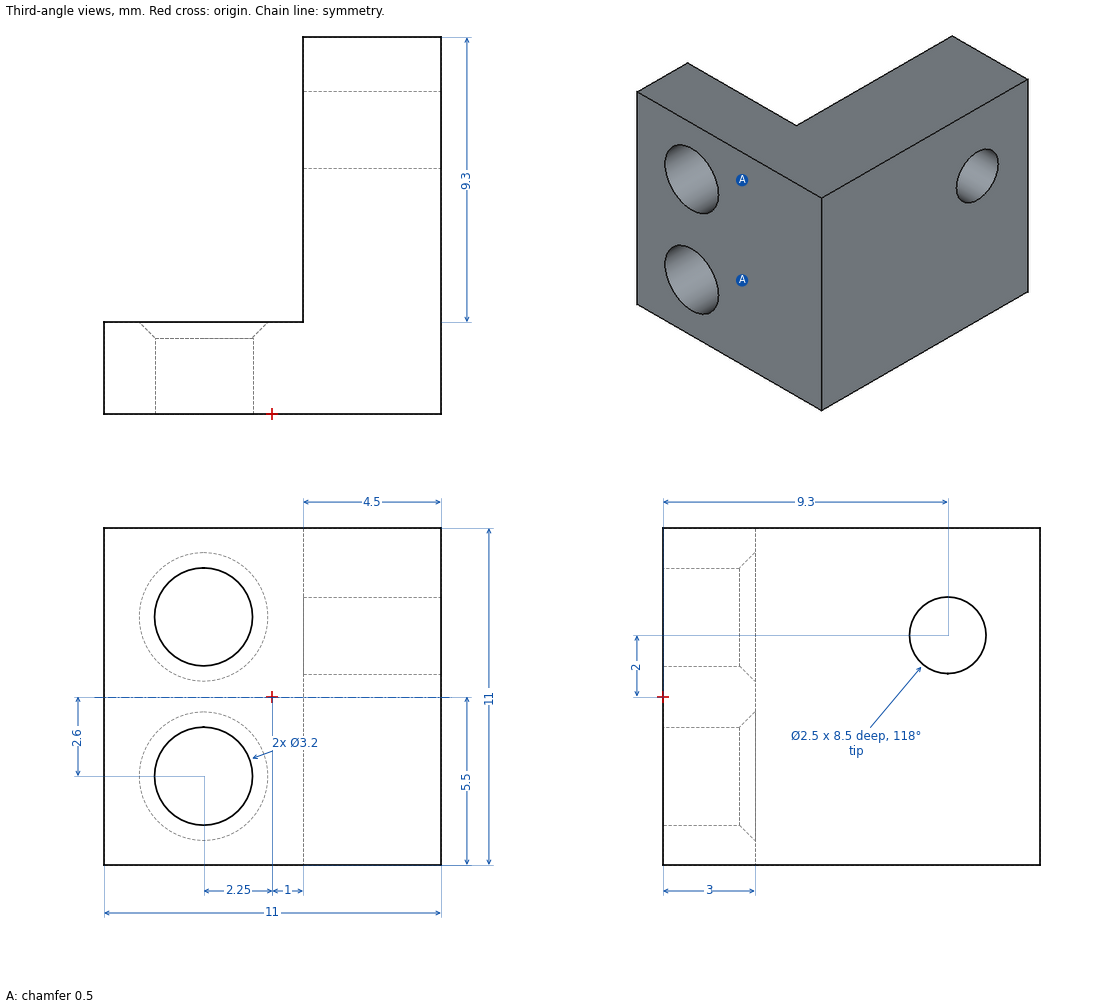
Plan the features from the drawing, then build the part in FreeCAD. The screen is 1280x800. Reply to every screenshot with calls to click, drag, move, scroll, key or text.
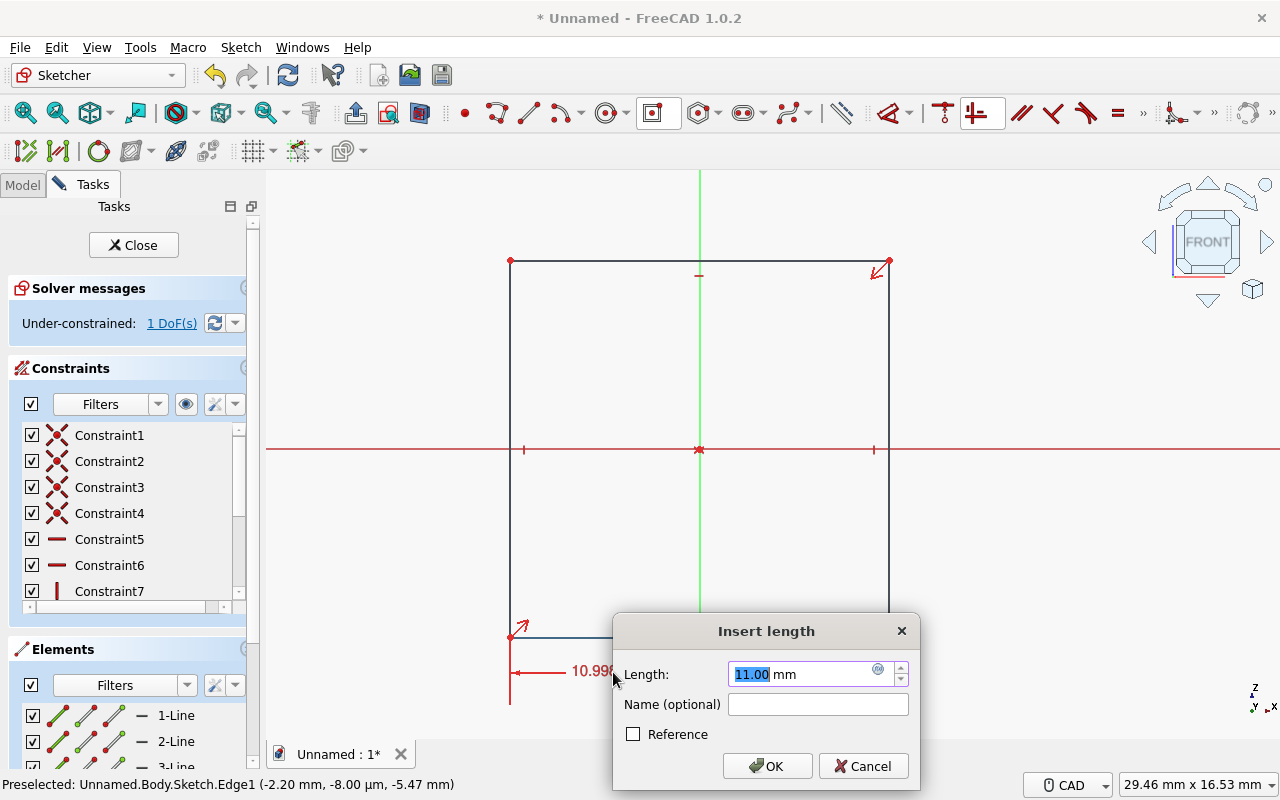
text(11)
key(Return)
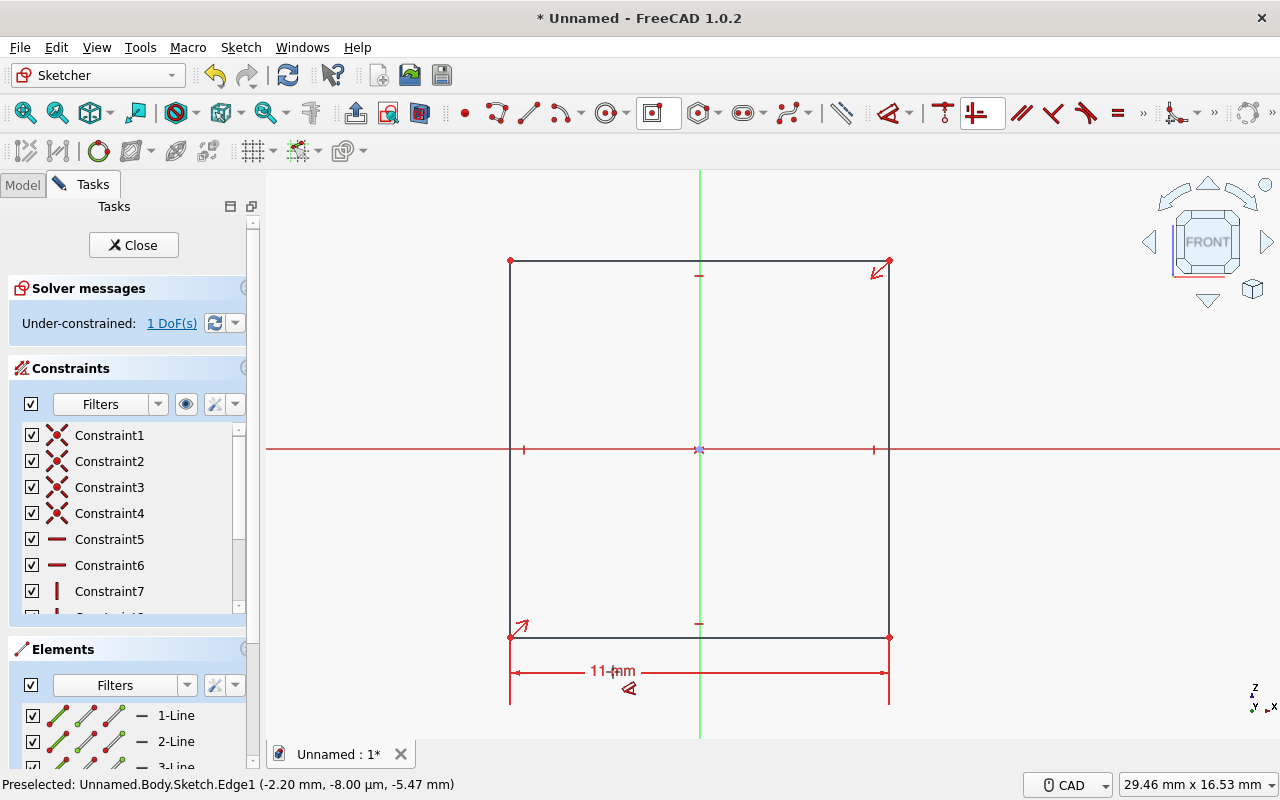
click(889, 525)
click(923, 363)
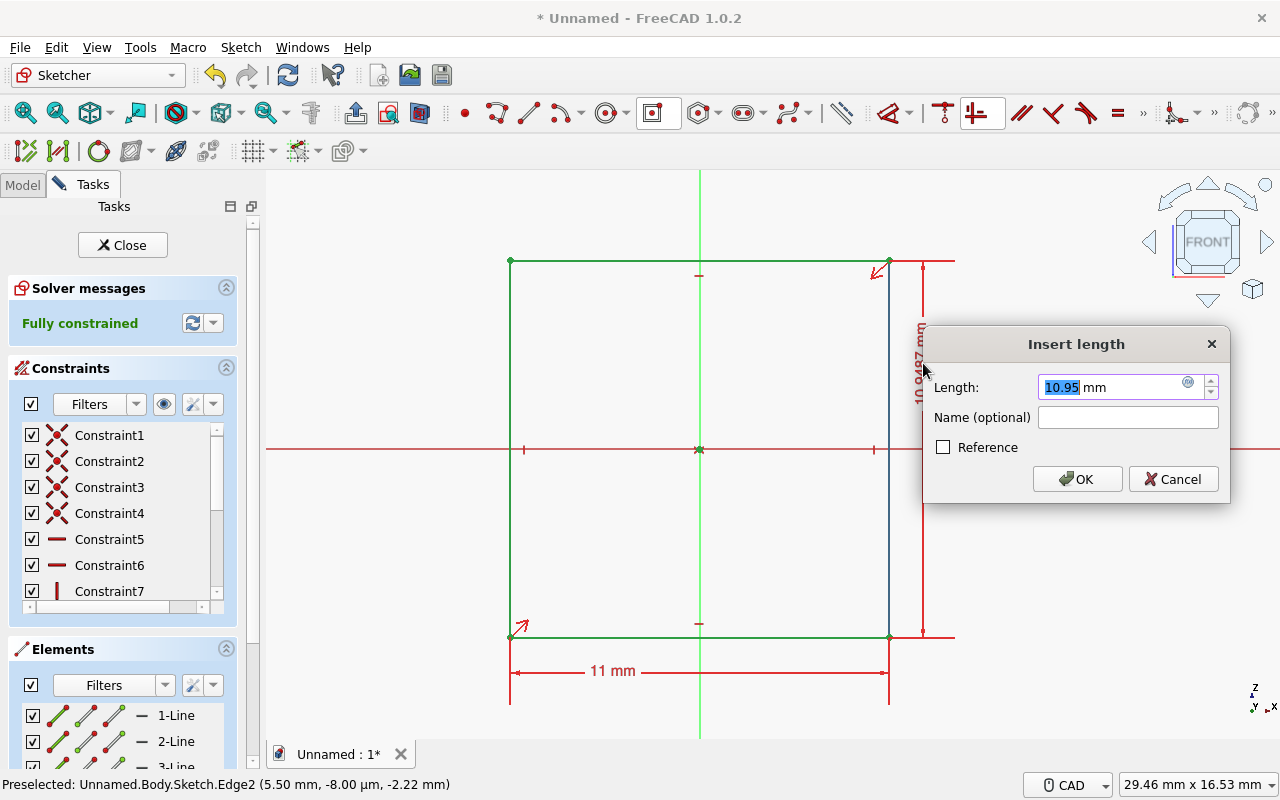
text(11)
key(Return)
key(Escape)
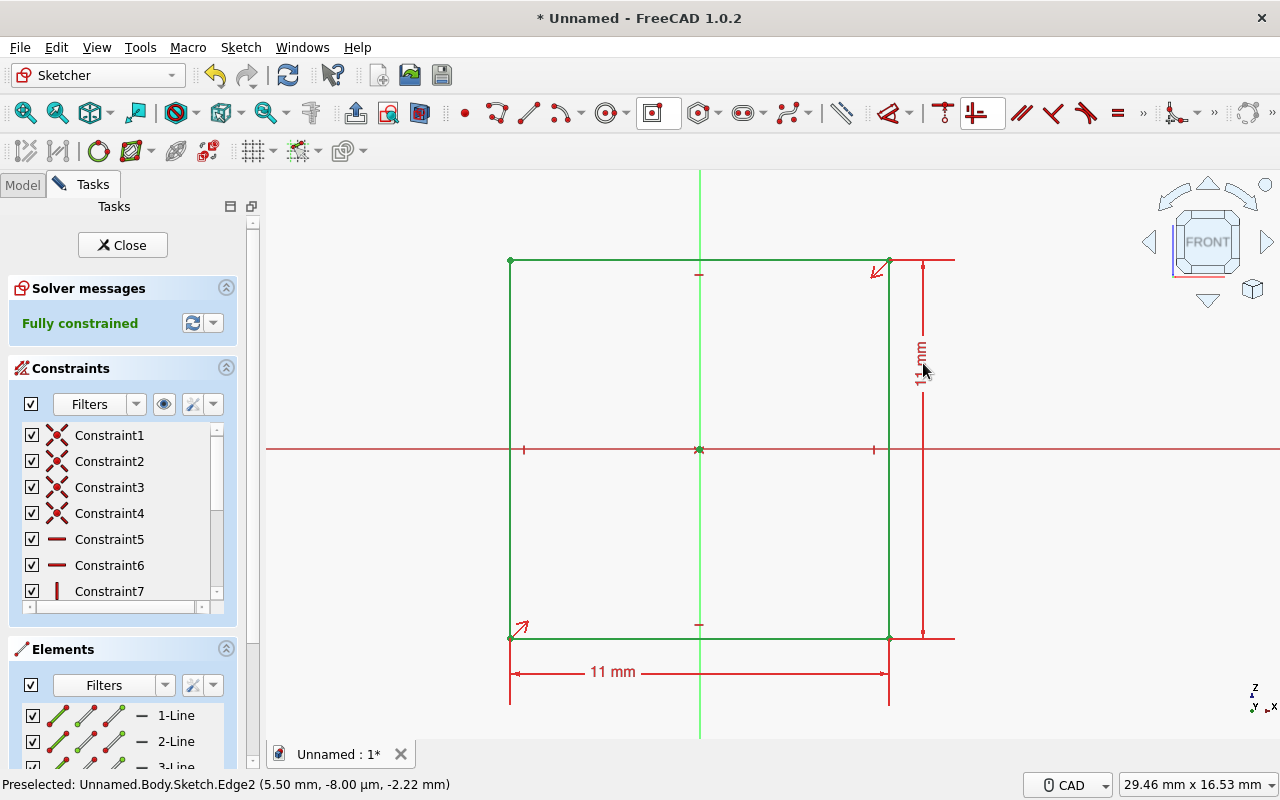
click(123, 245)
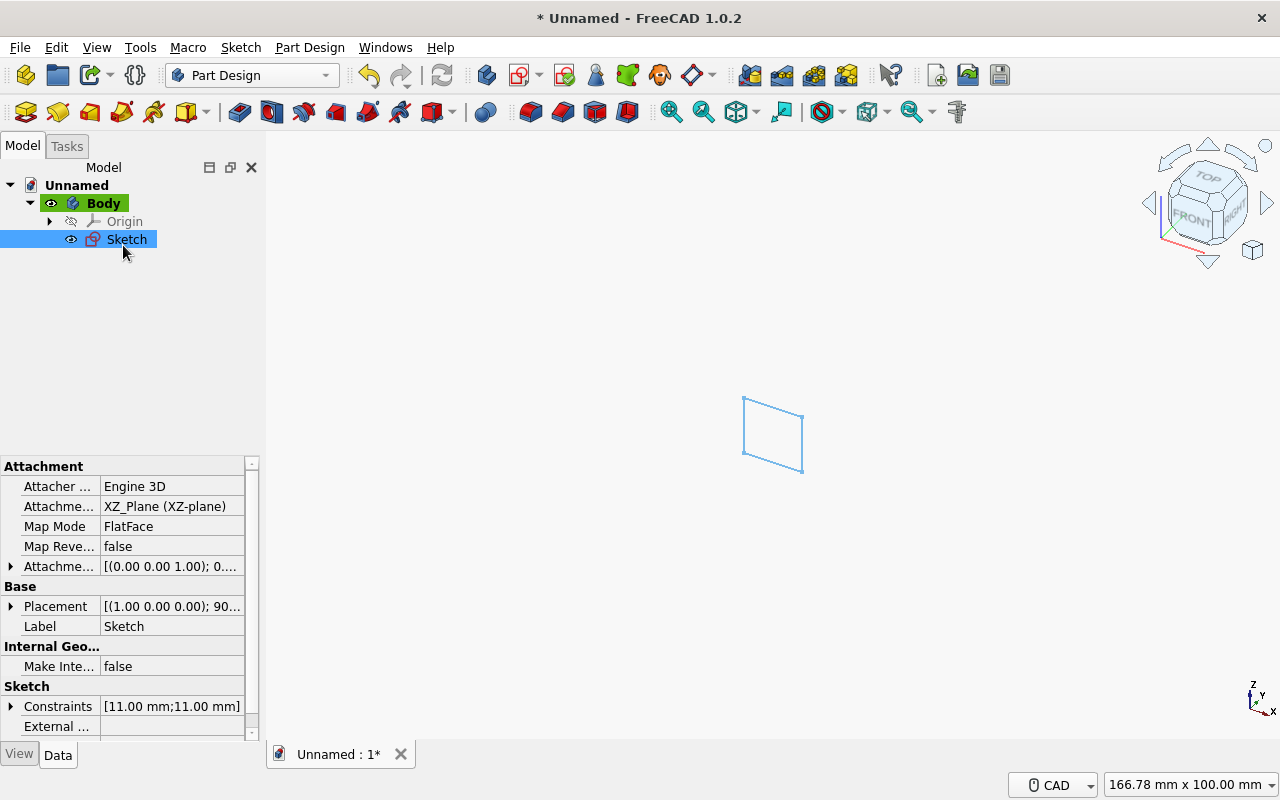
click(26, 112)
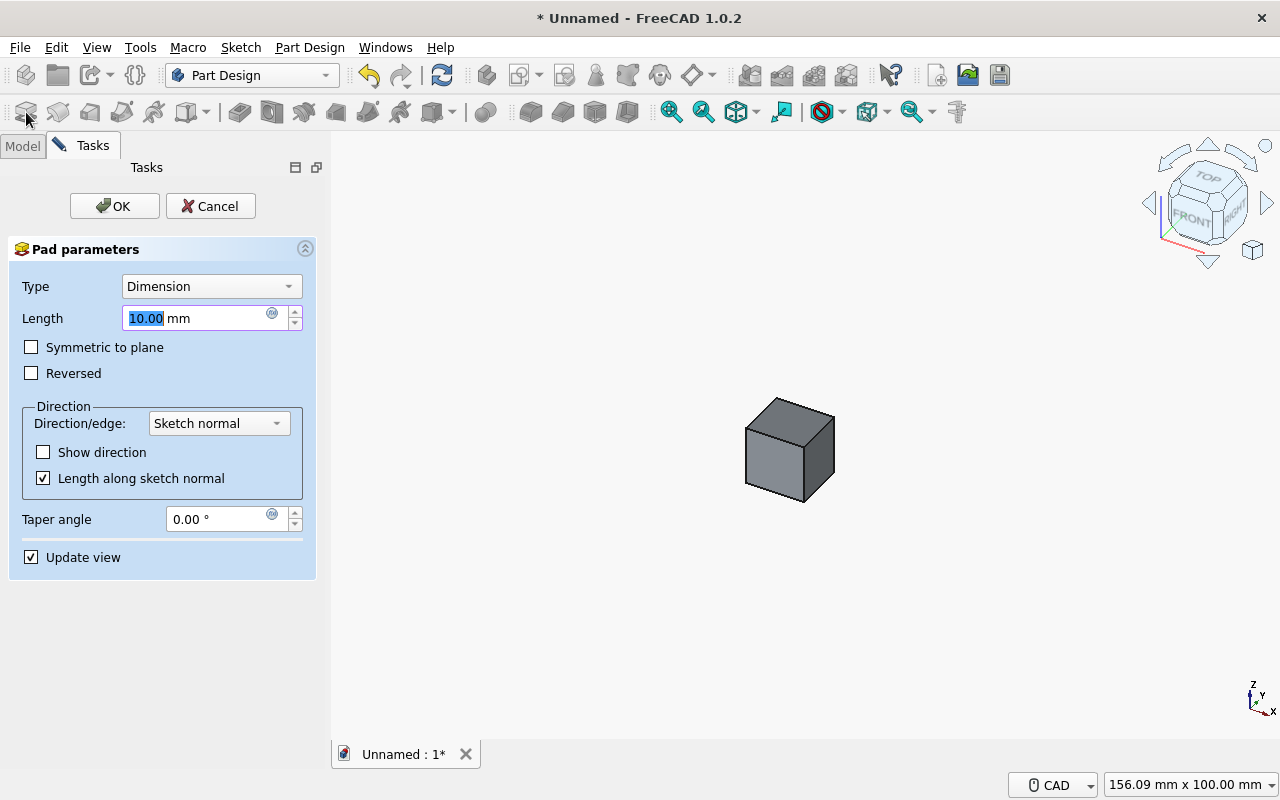
text(3)
key(Tab)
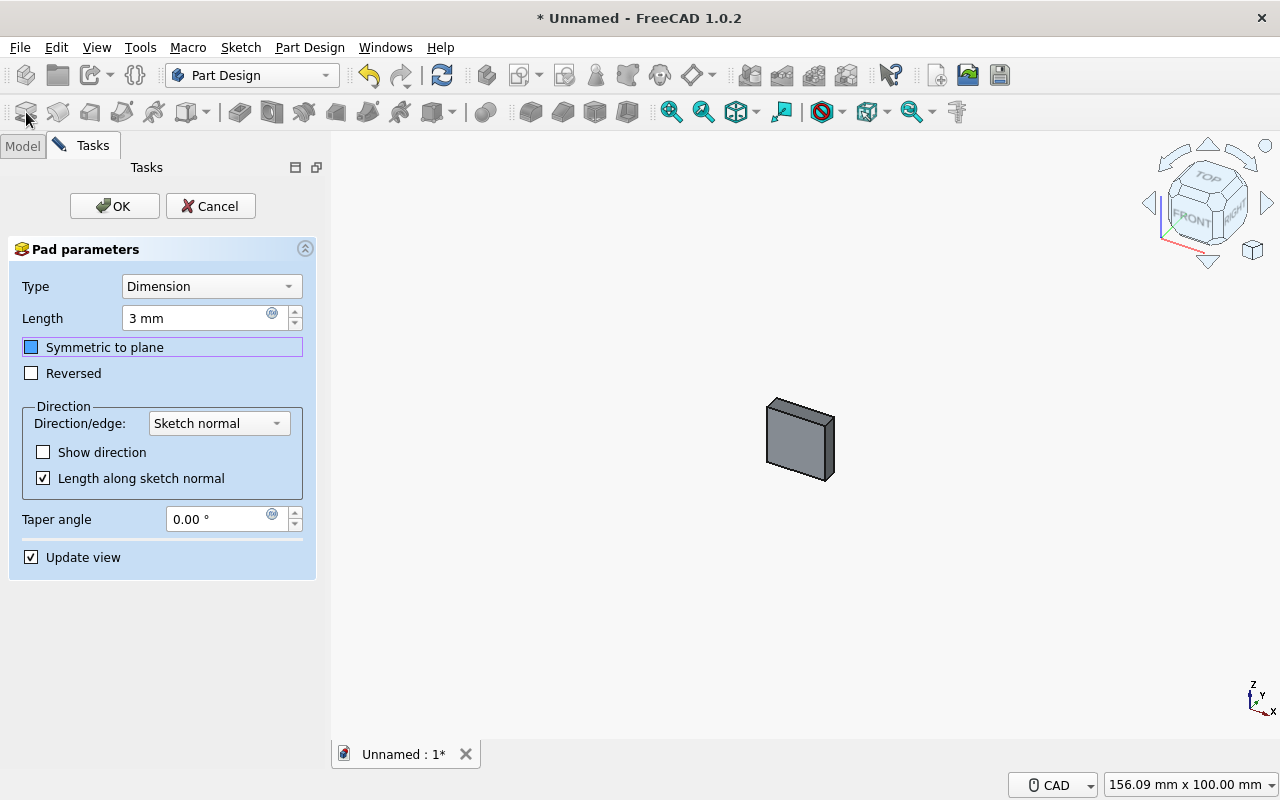
click(30, 373)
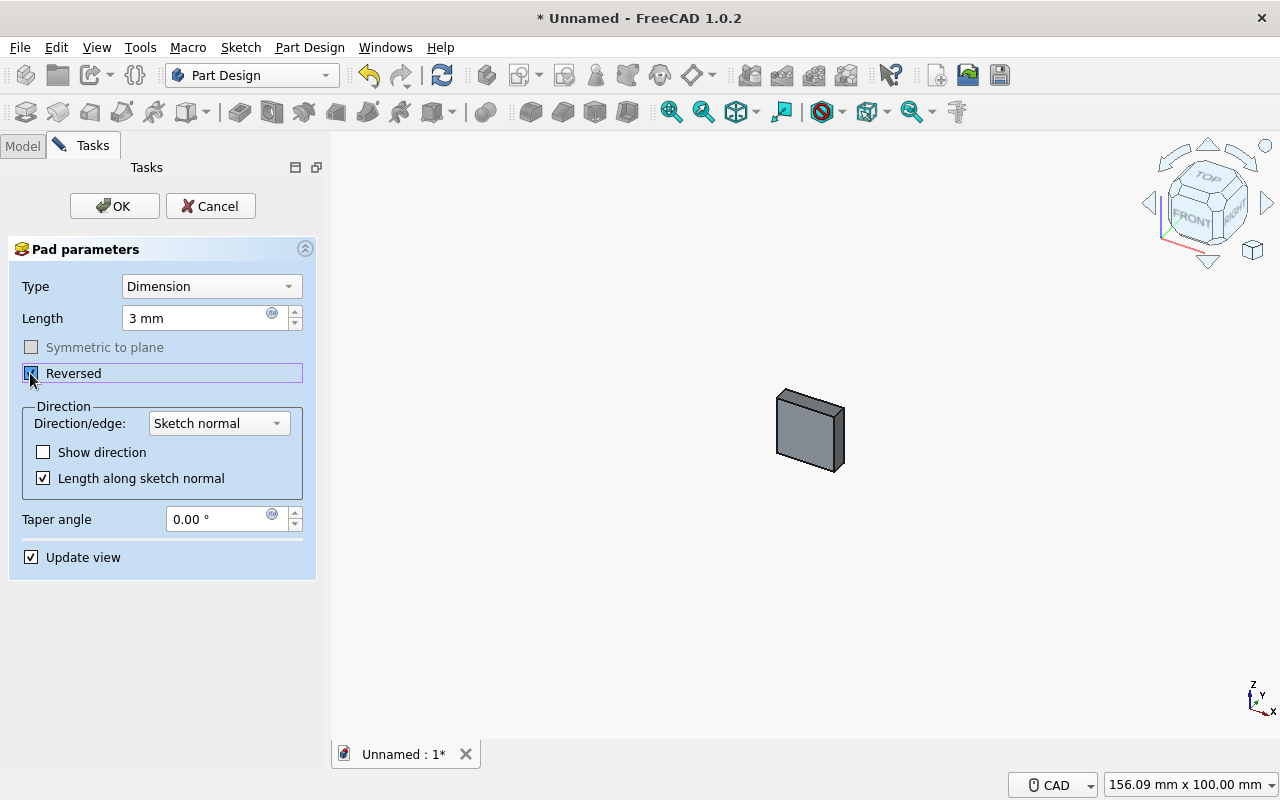
click(115, 206)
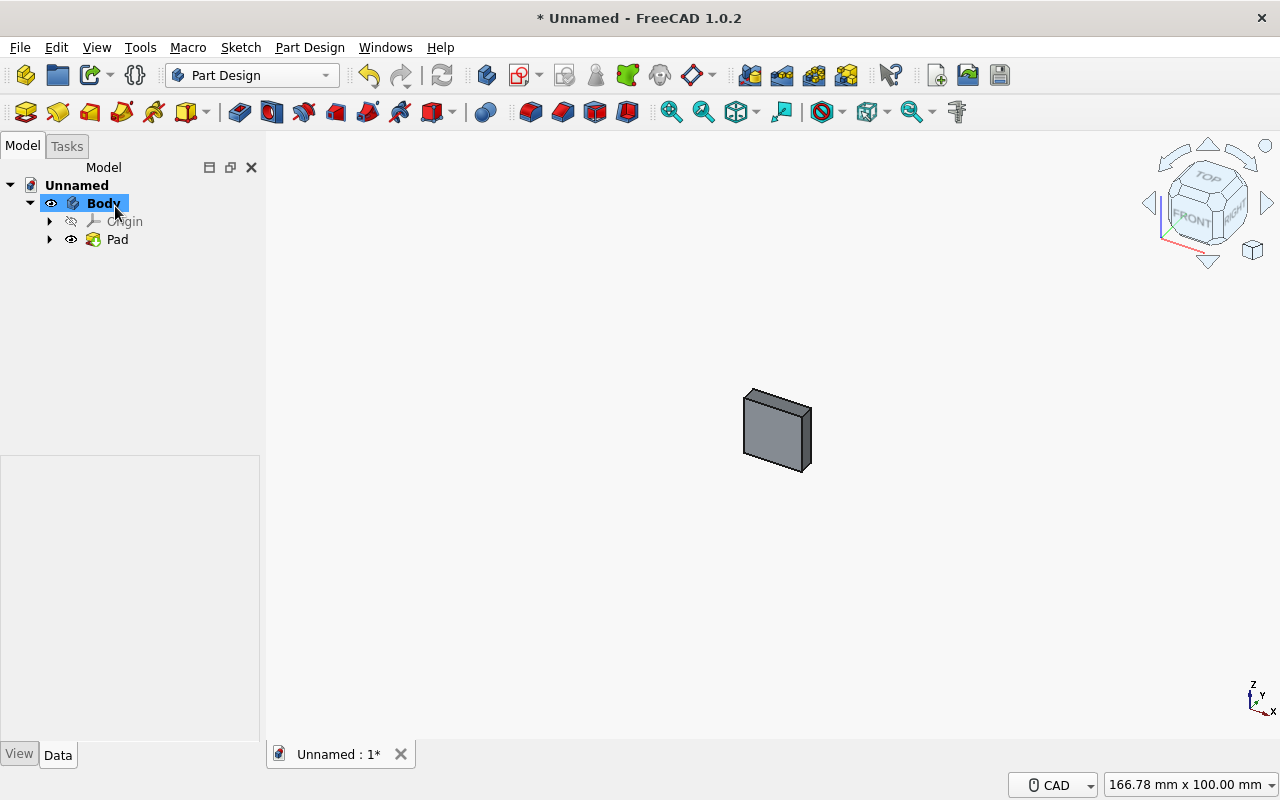
click(672, 112)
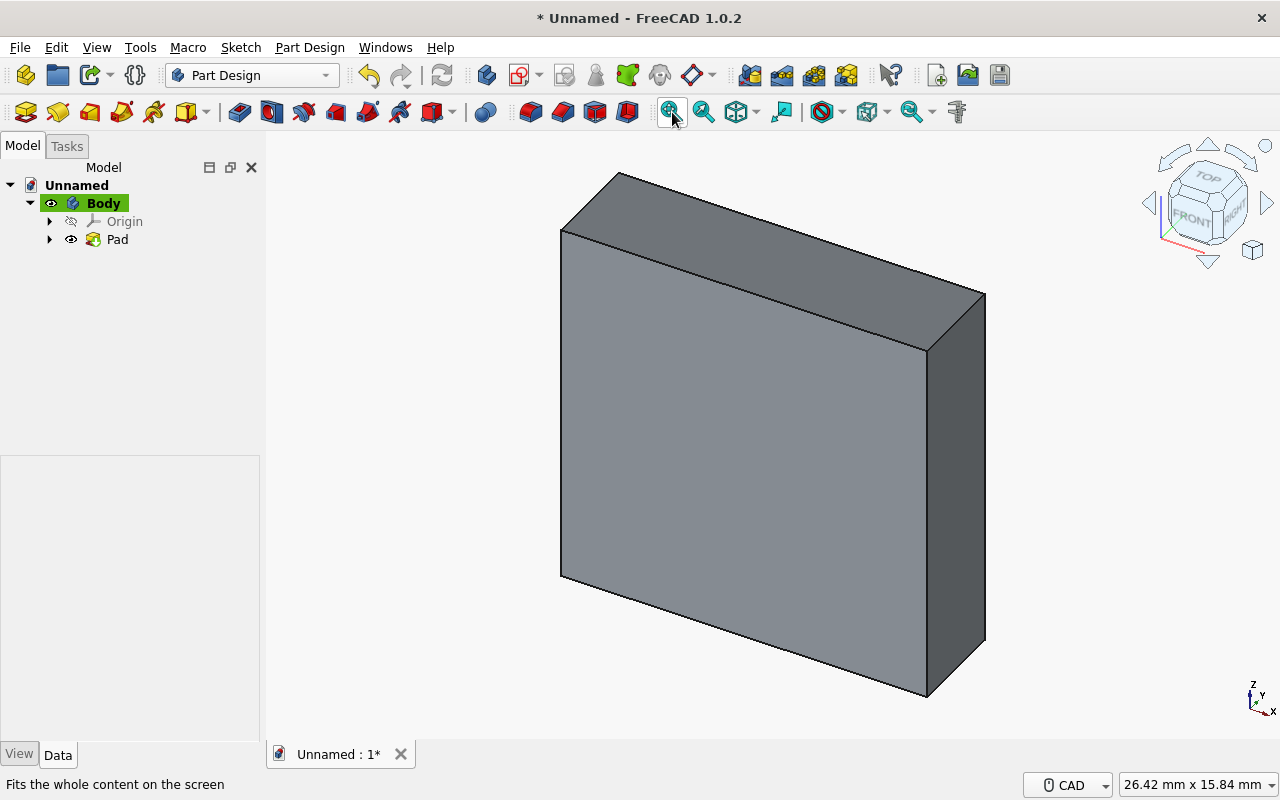
key(4)